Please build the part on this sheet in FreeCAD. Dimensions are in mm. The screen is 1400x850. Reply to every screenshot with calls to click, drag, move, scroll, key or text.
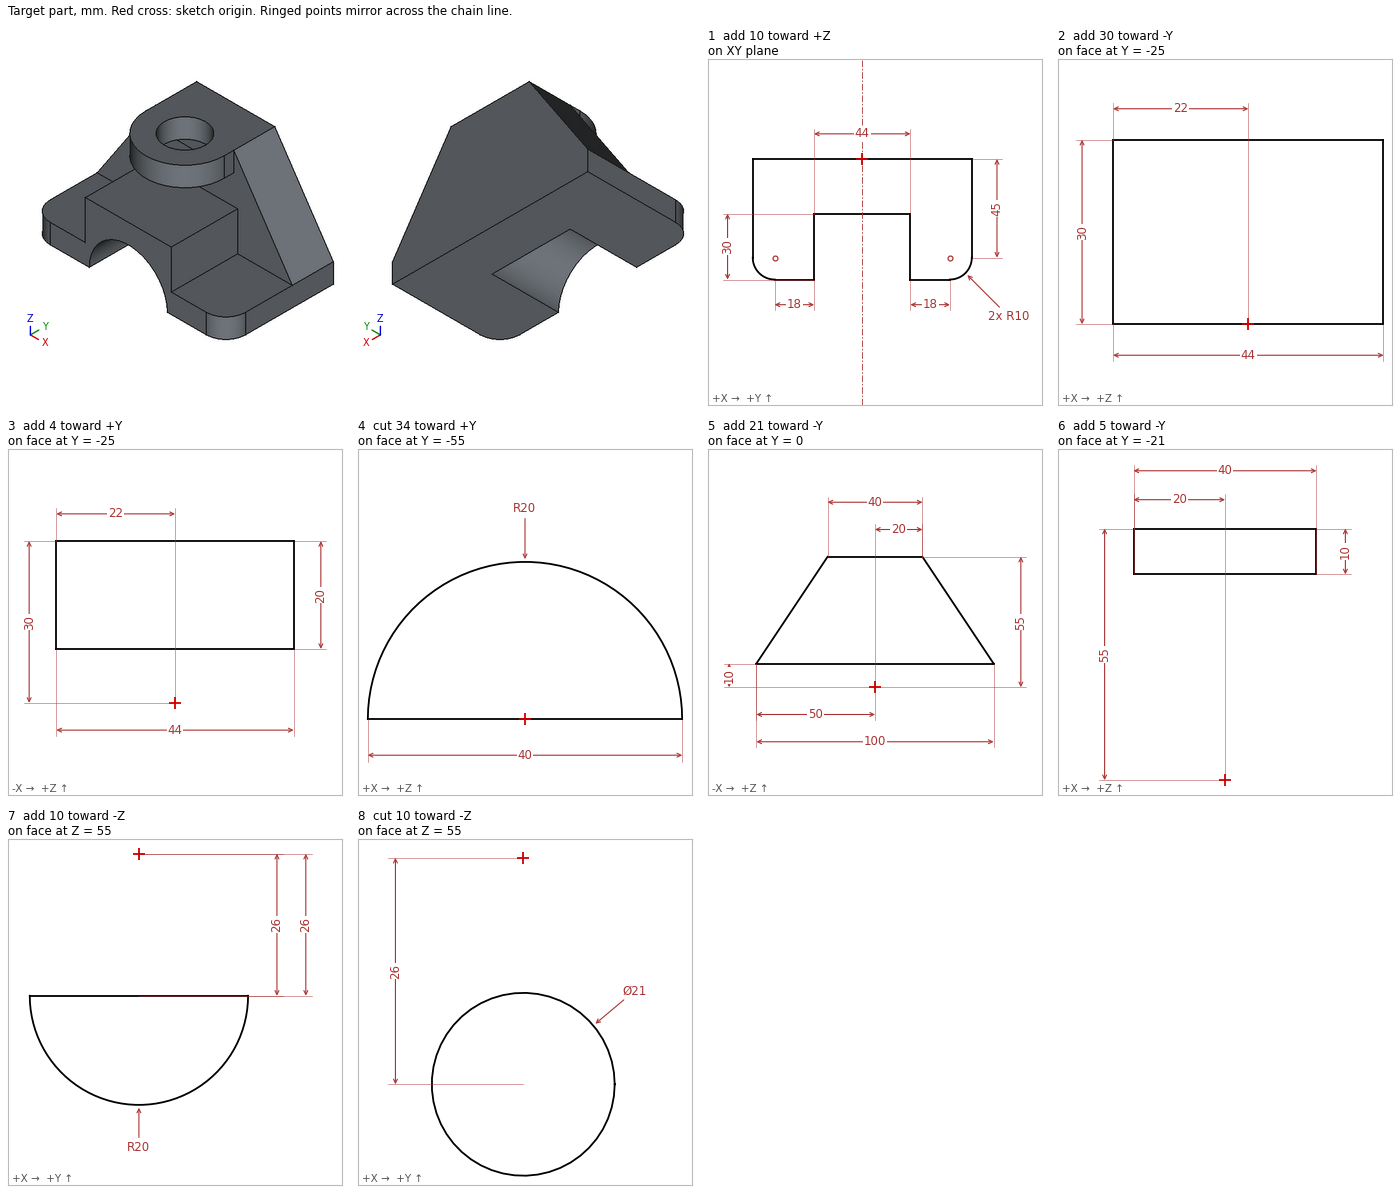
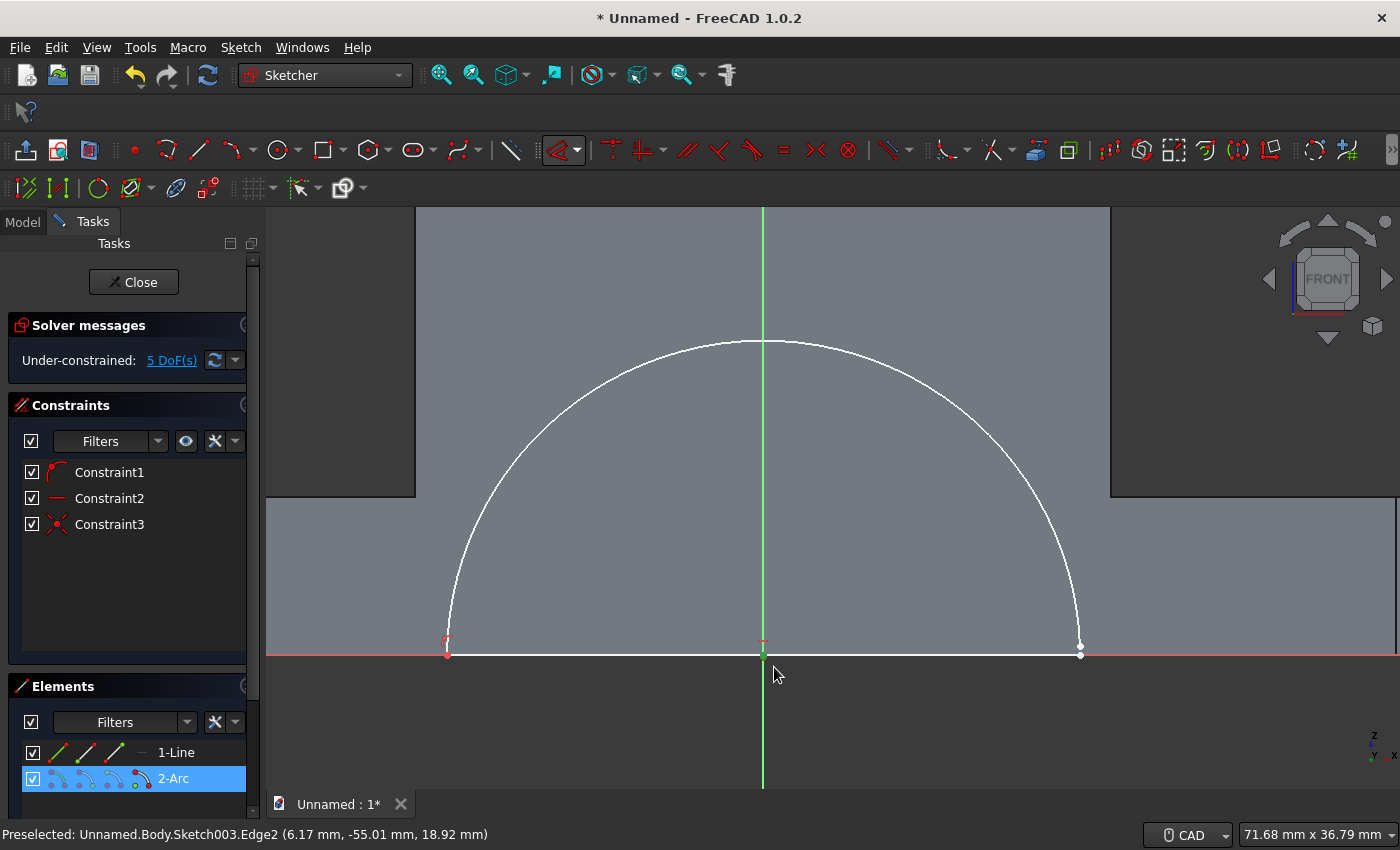
click(612, 150)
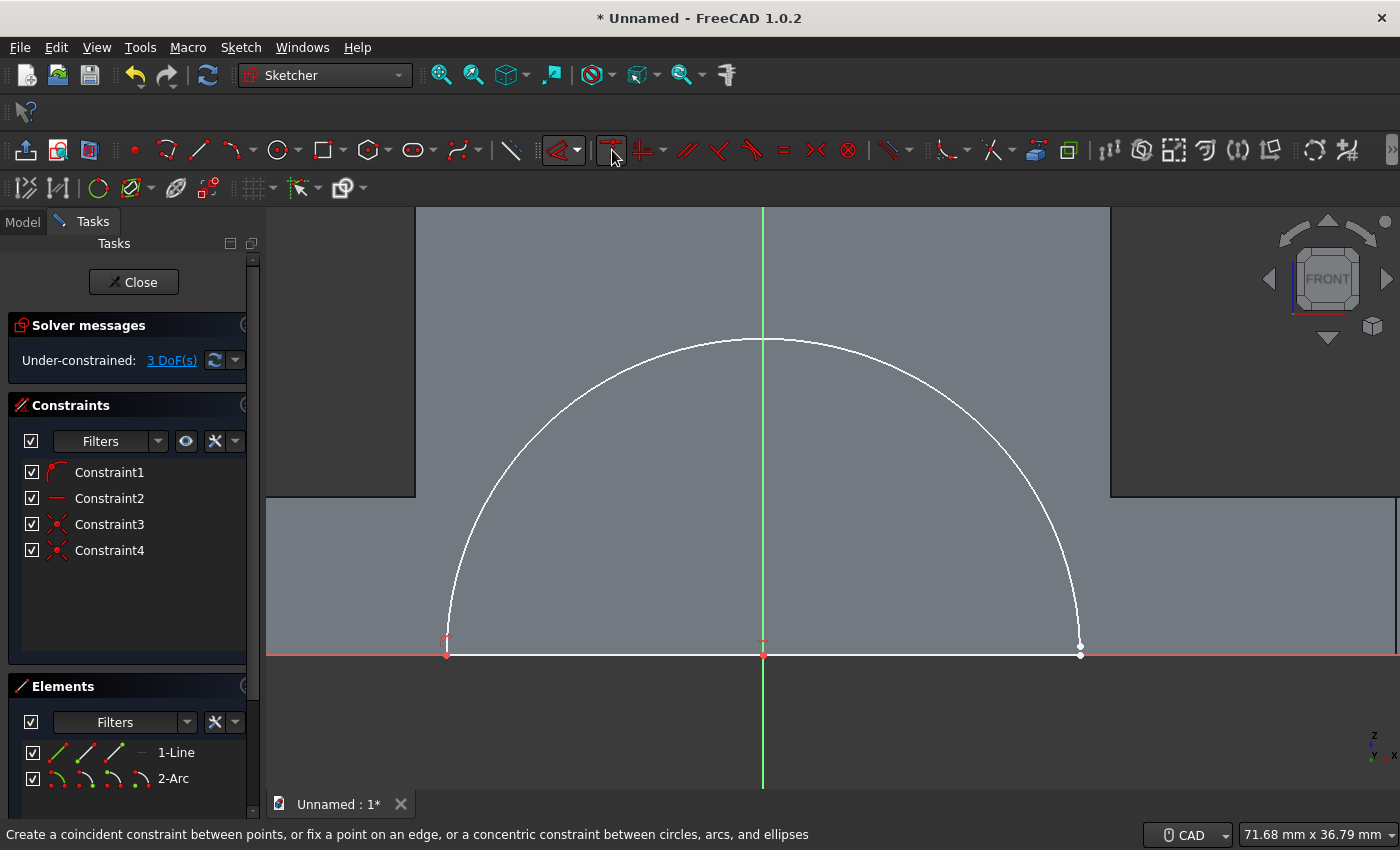
click(945, 396)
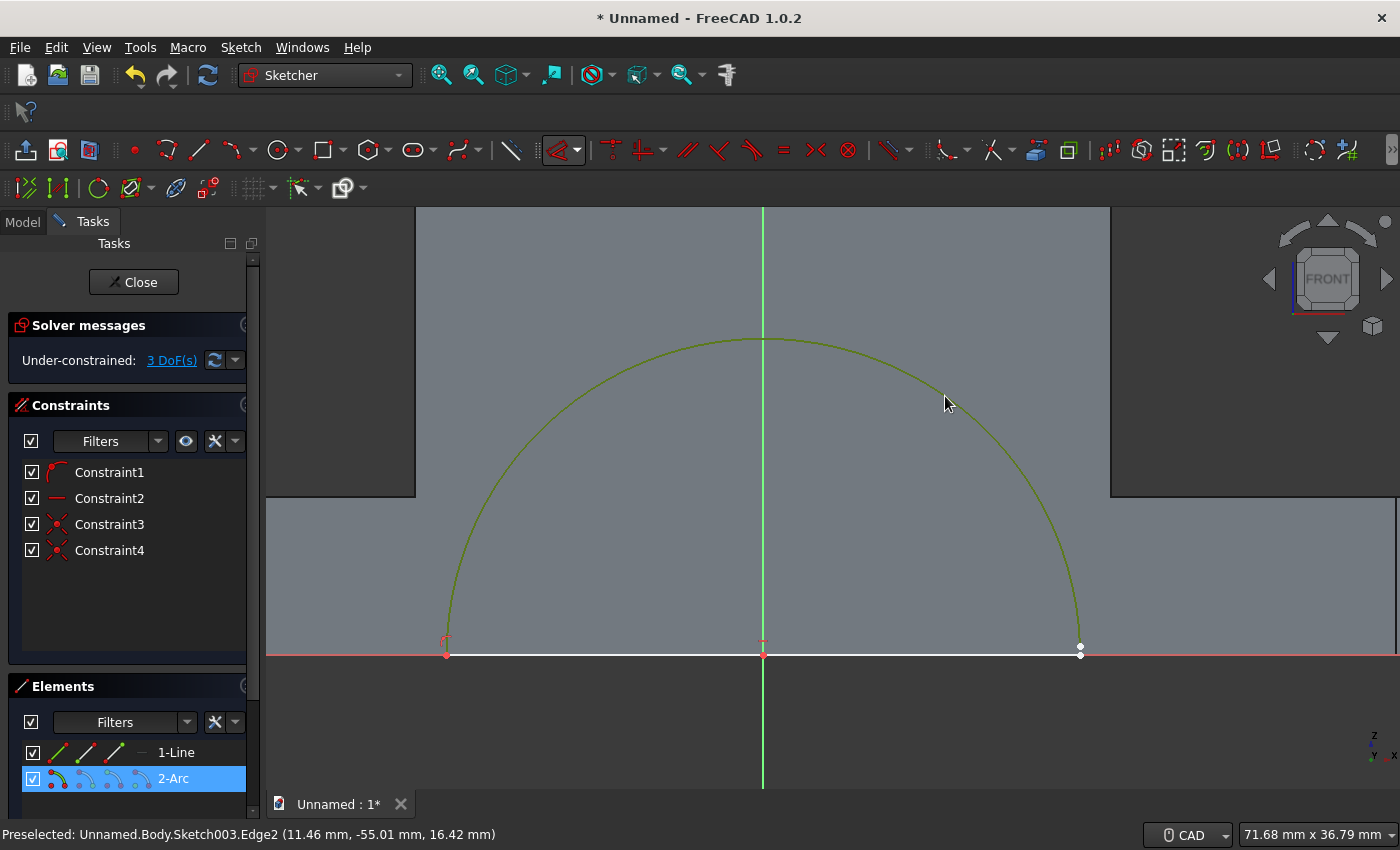
key(k)
key(r)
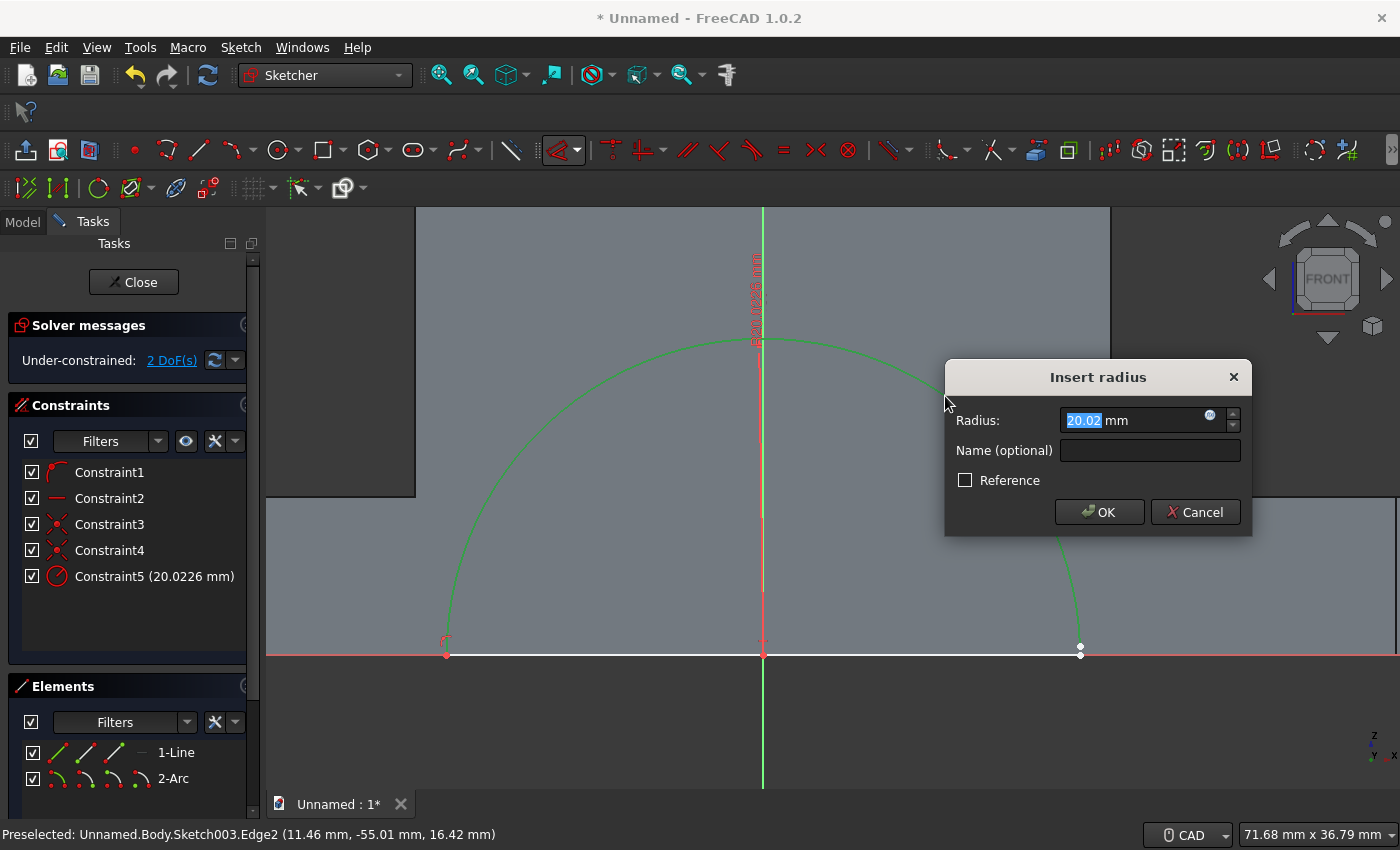
text(20)
key(Return)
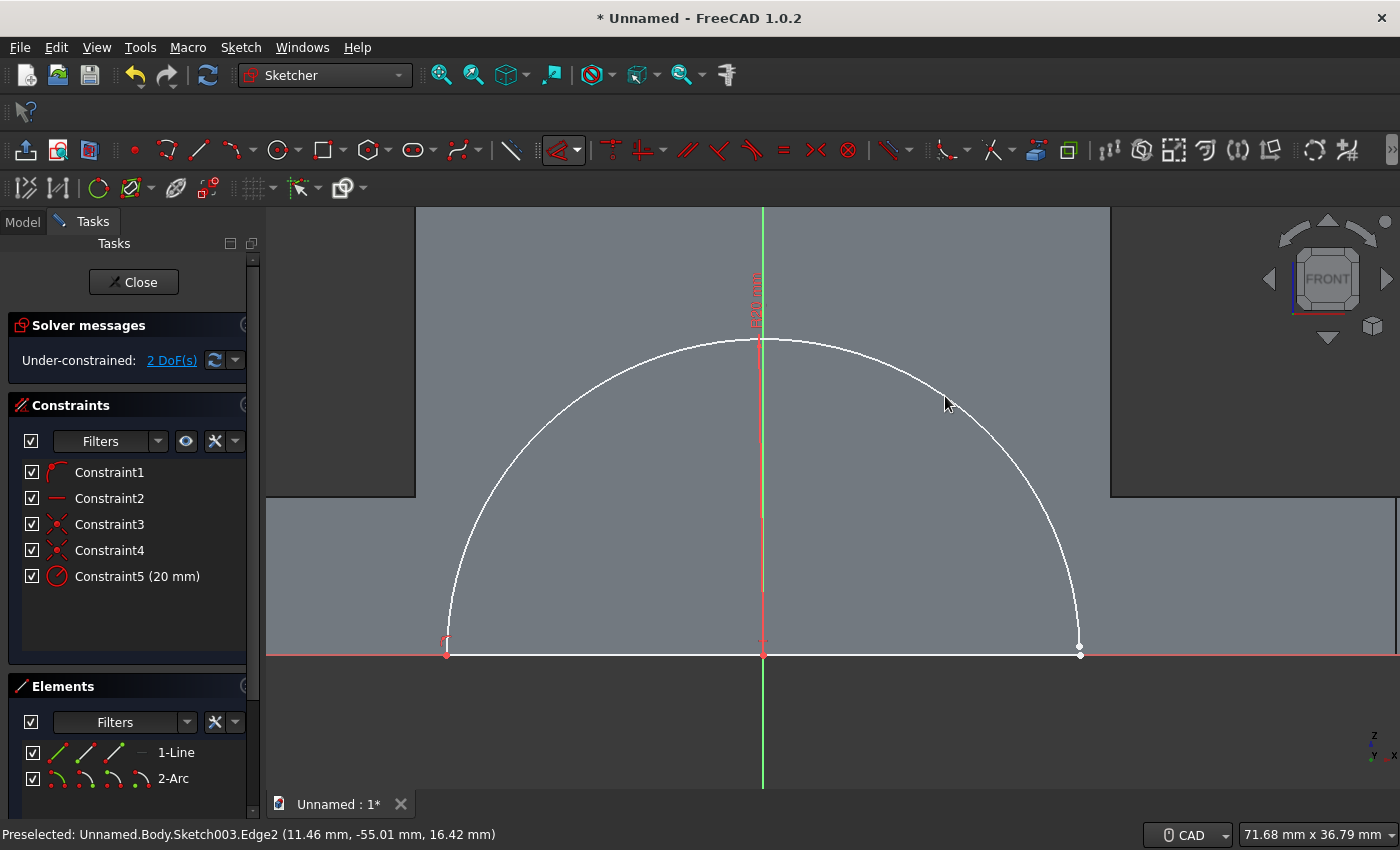
click(1080, 647)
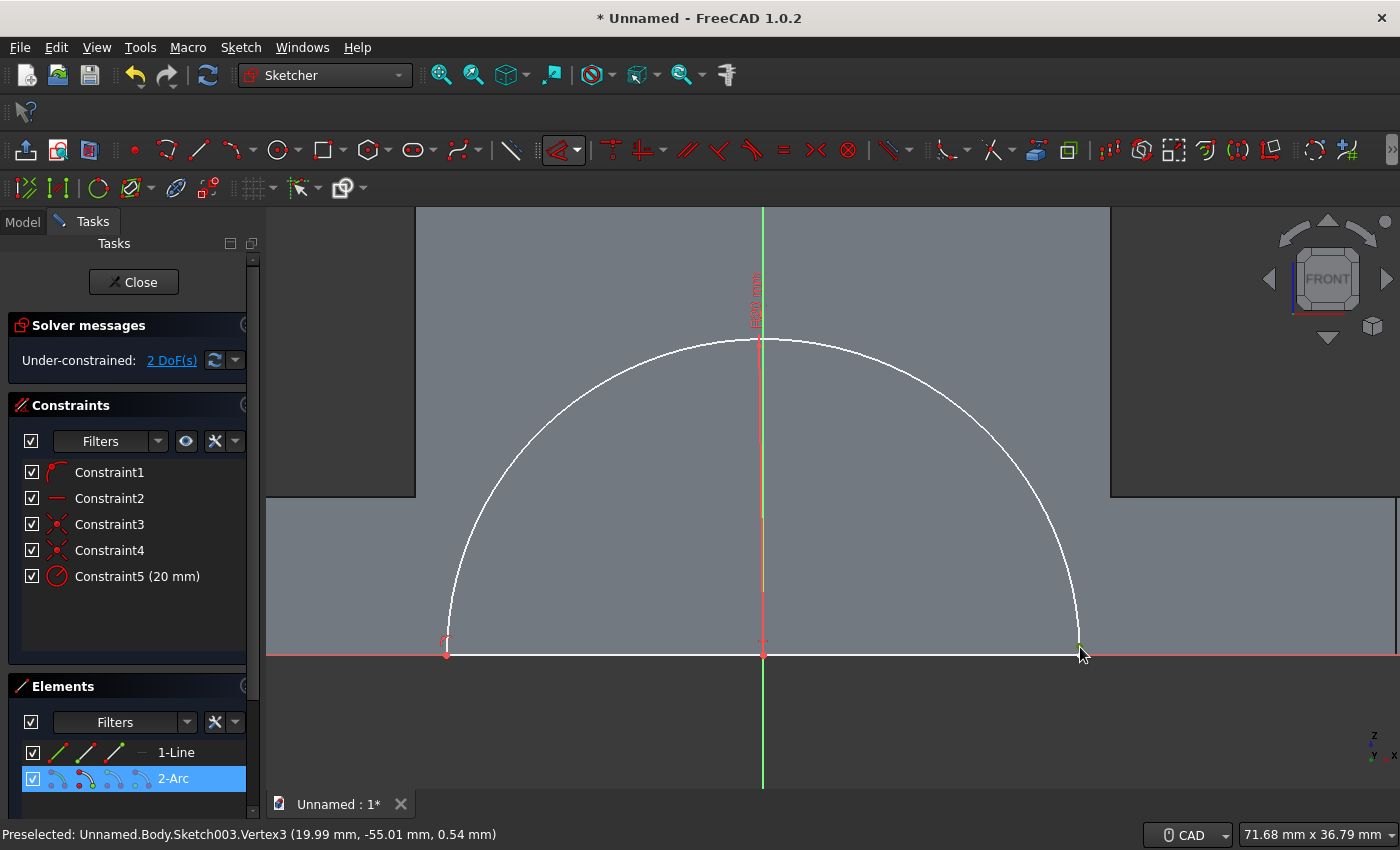
click(361, 655)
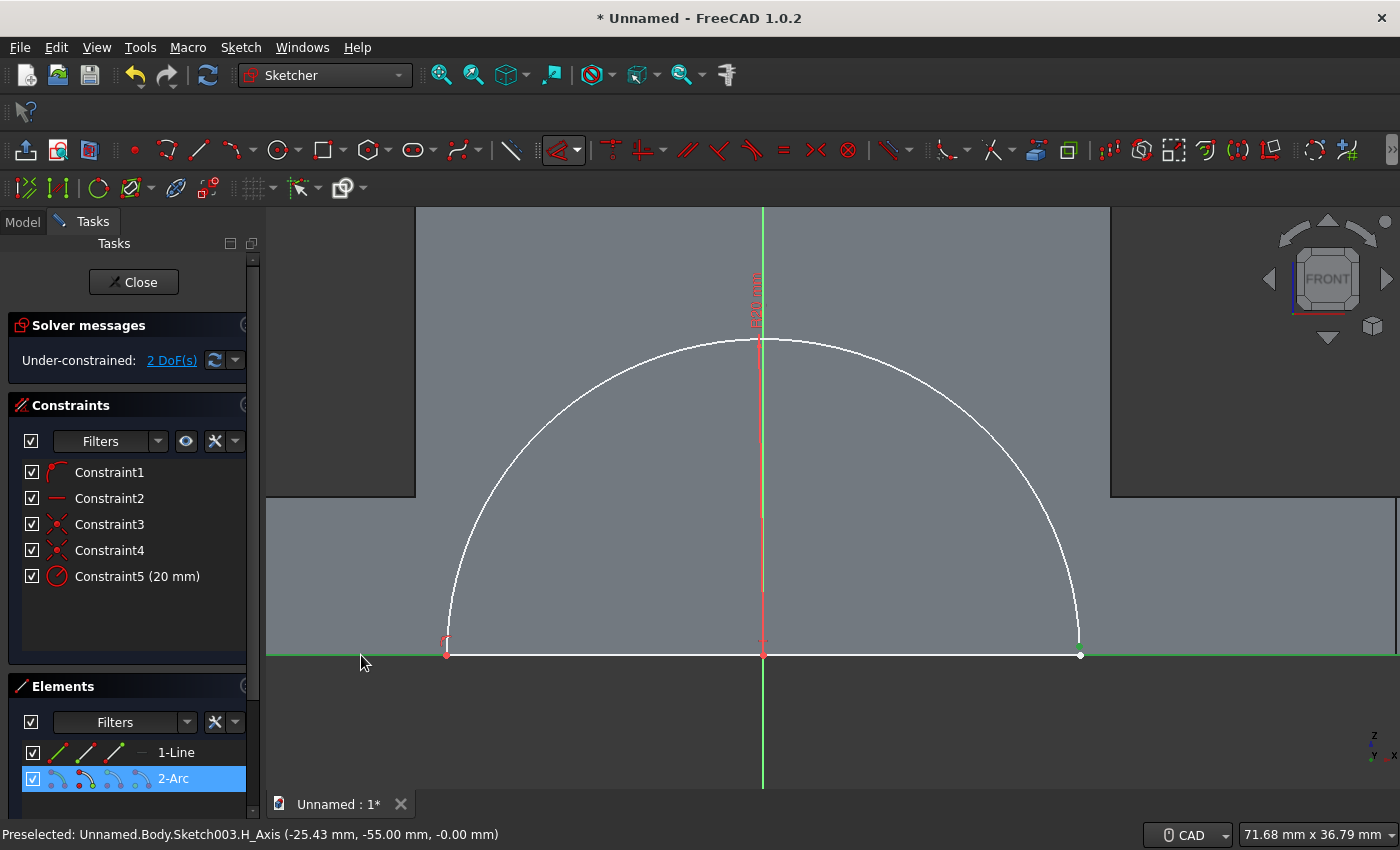
click(612, 150)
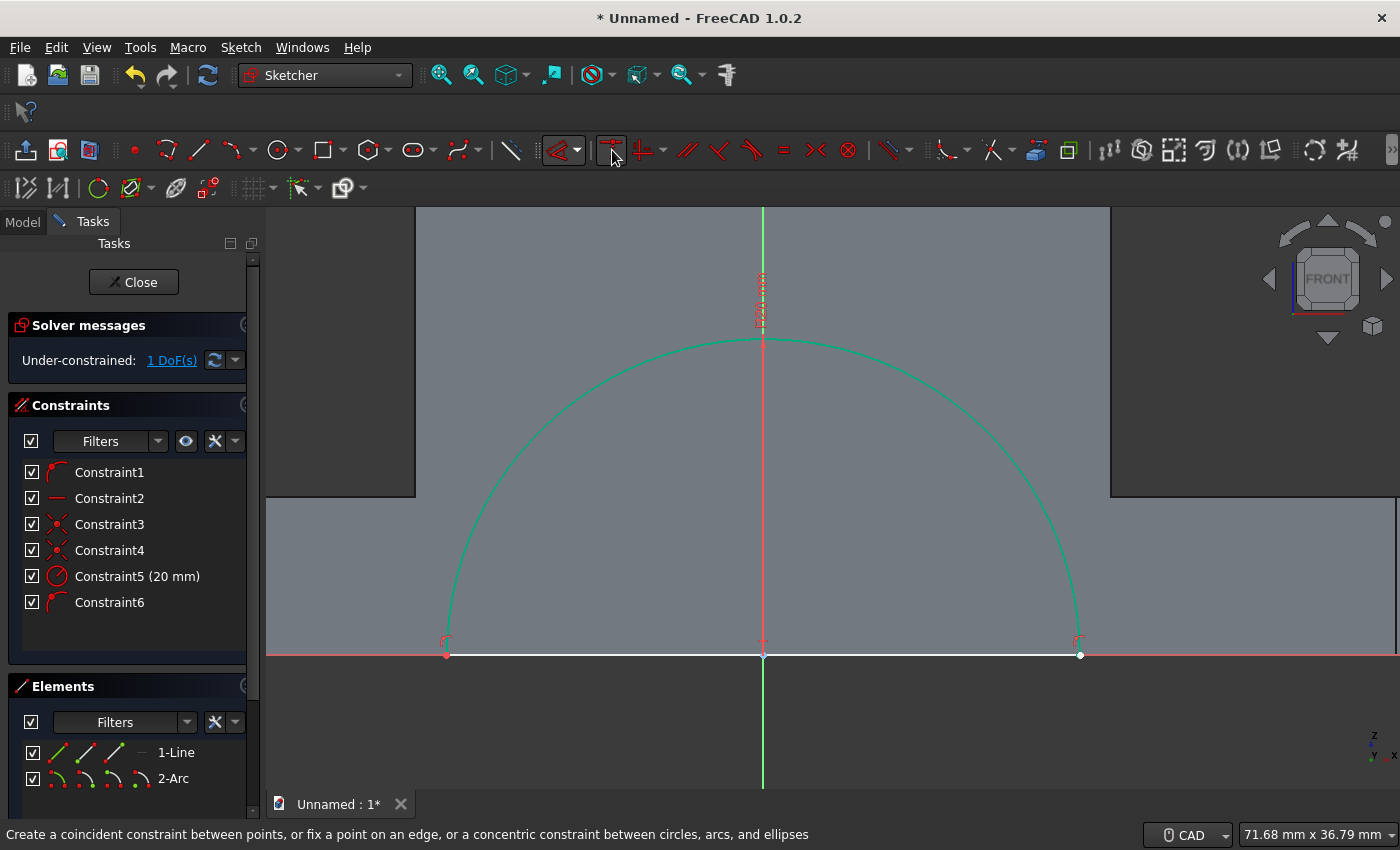
click(637, 655)